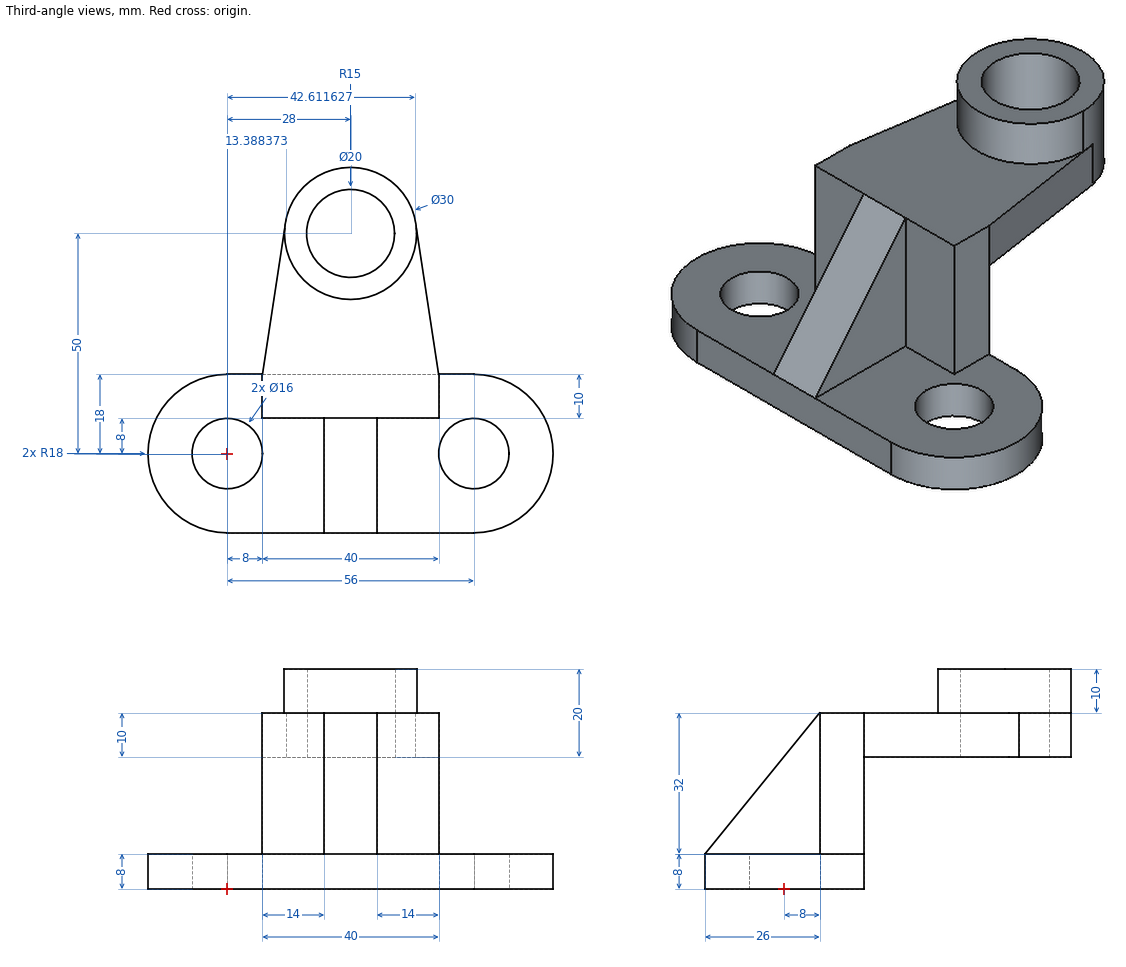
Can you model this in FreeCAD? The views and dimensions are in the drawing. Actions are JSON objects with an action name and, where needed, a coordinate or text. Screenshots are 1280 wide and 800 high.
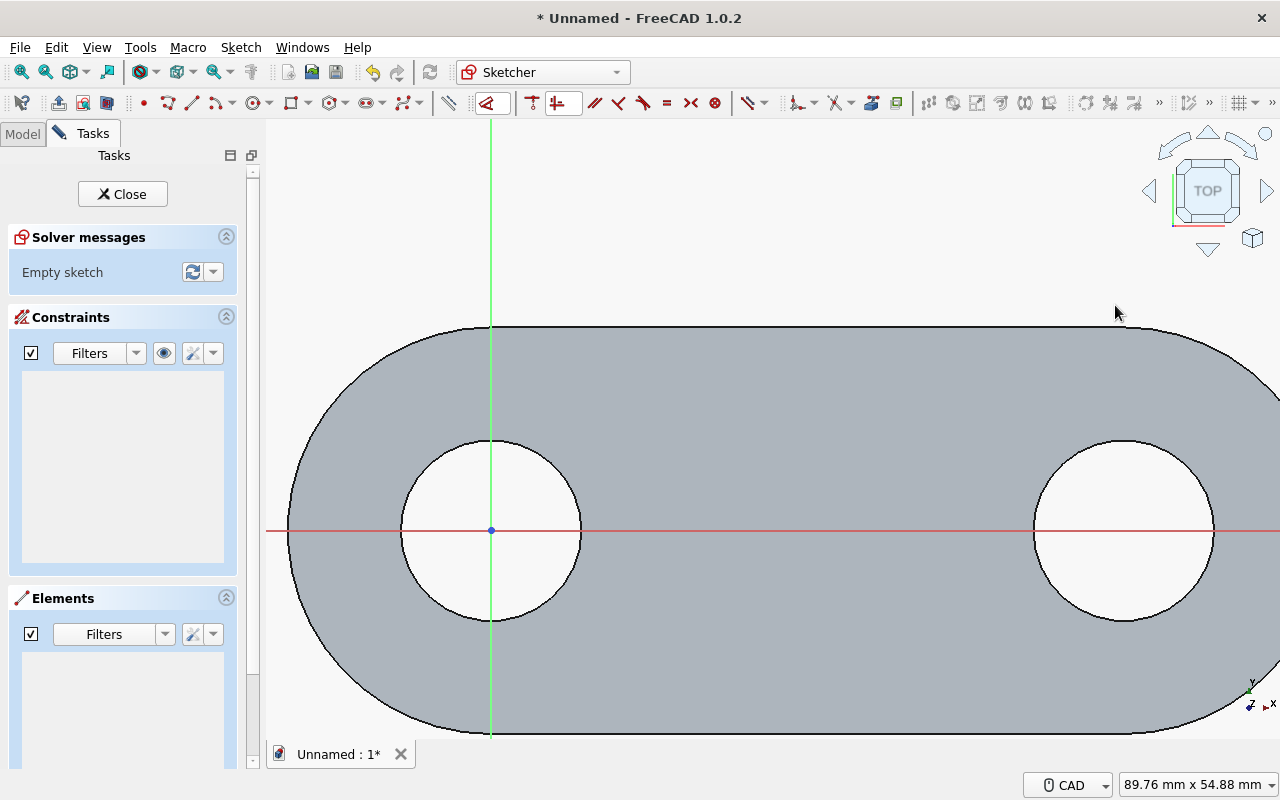
{"action": "left_click", "coordinate": [292, 104]}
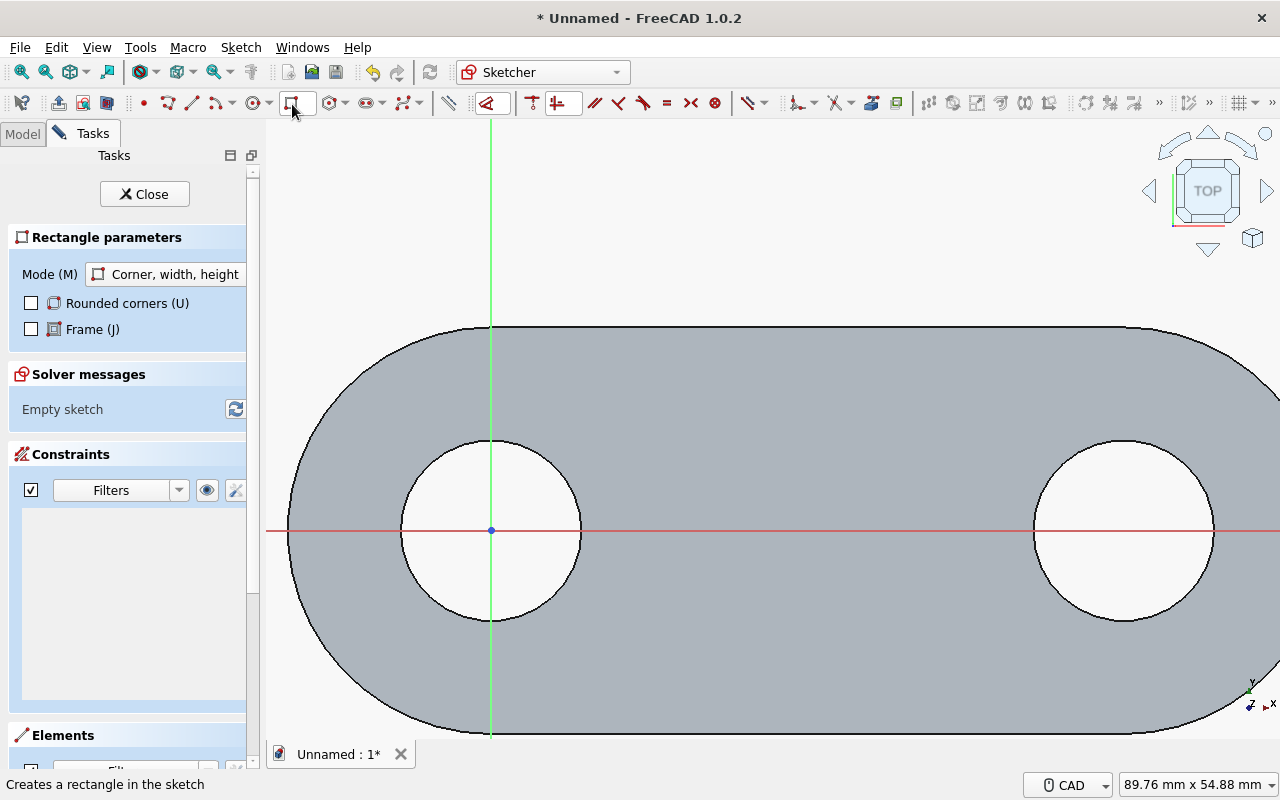
{"action": "left_click", "coordinate": [582, 327]}
{"action": "mouse_move", "coordinate": [1033, 440]}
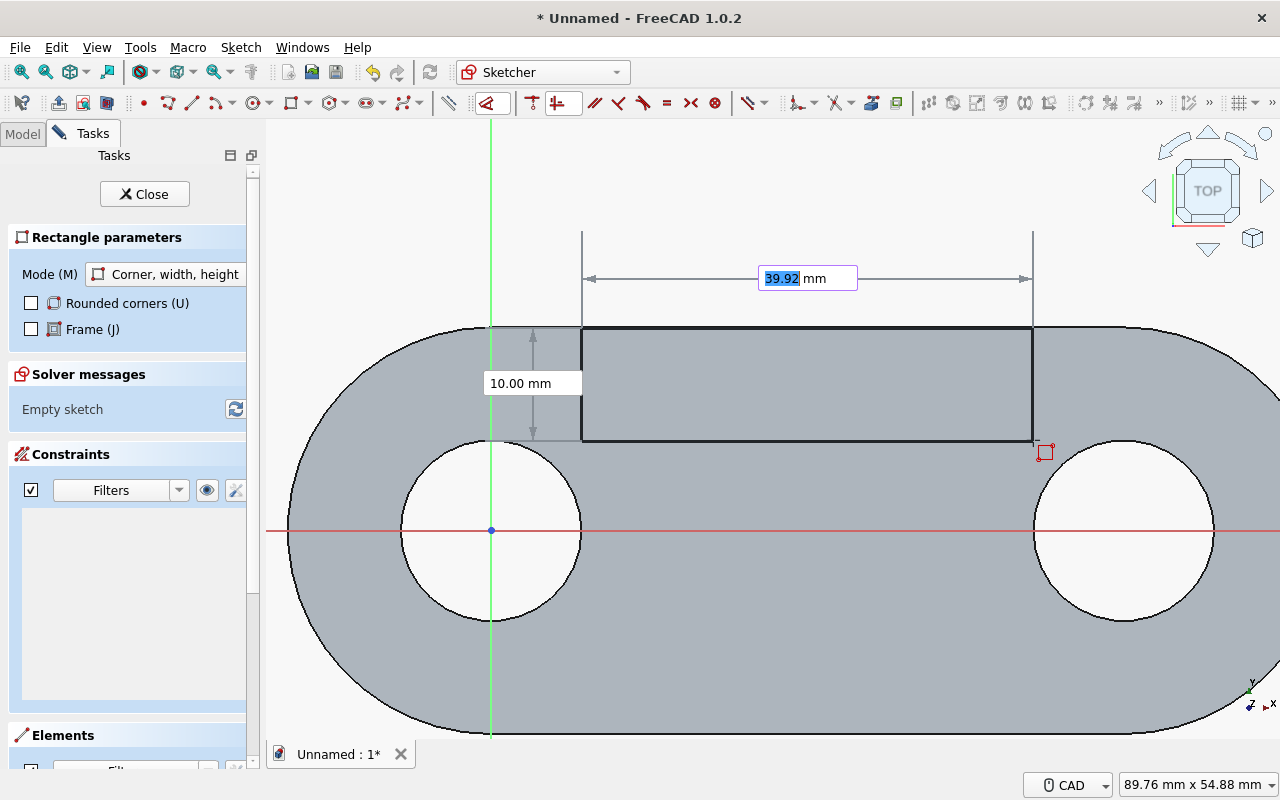
{"action": "type", "text": "40"}
{"action": "key", "text": "Tab"}
{"action": "type", "text": "10"}
{"action": "key", "text": "Return"}
{"action": "key", "text": "Escape"}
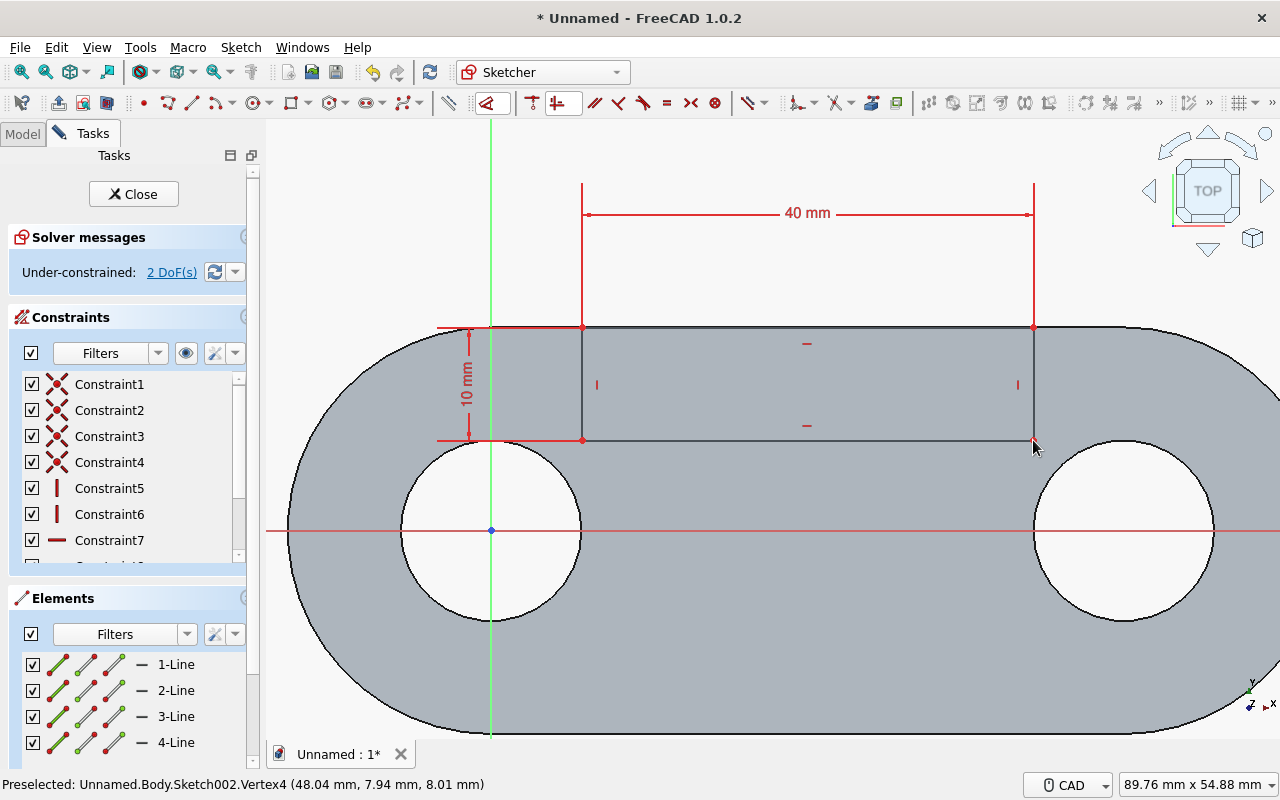
{"action": "left_click", "coordinate": [582, 328]}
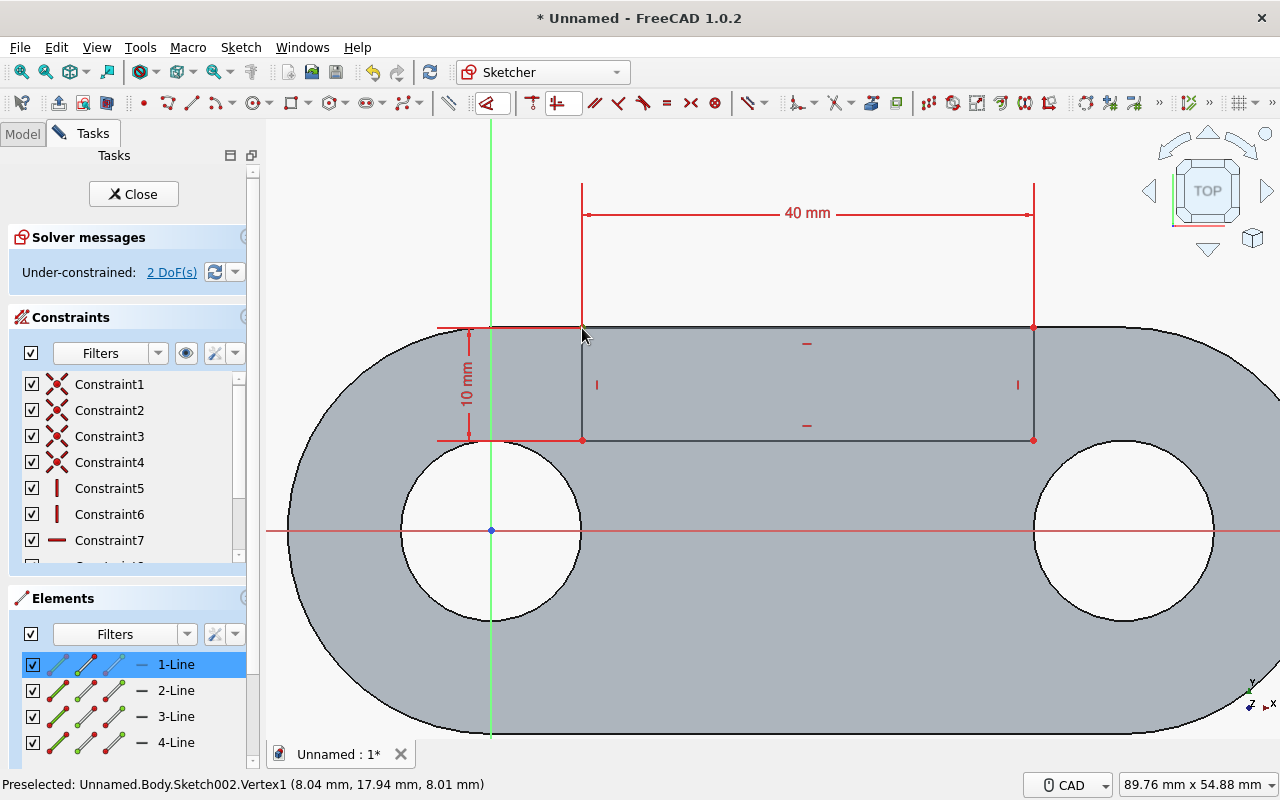
{"action": "key", "text": "l"}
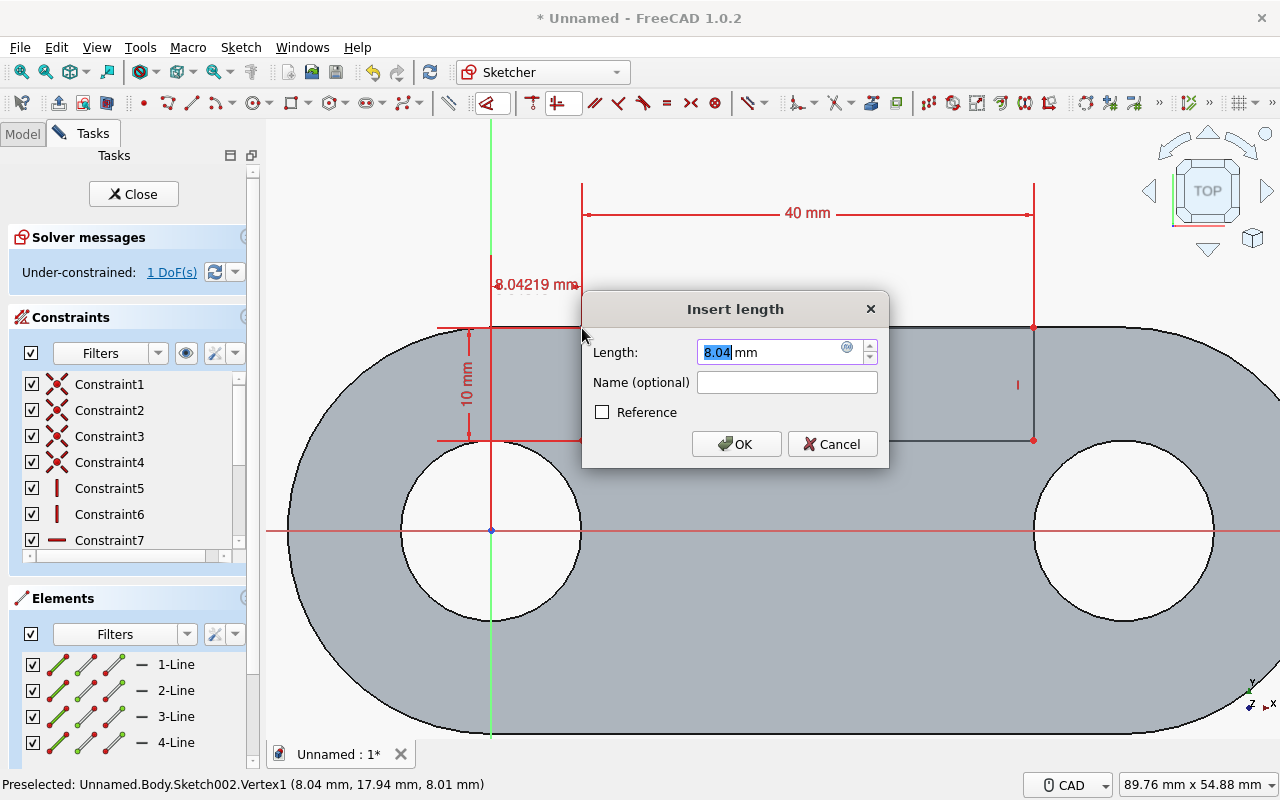
{"action": "type", "text": "8"}
{"action": "key", "text": "Return"}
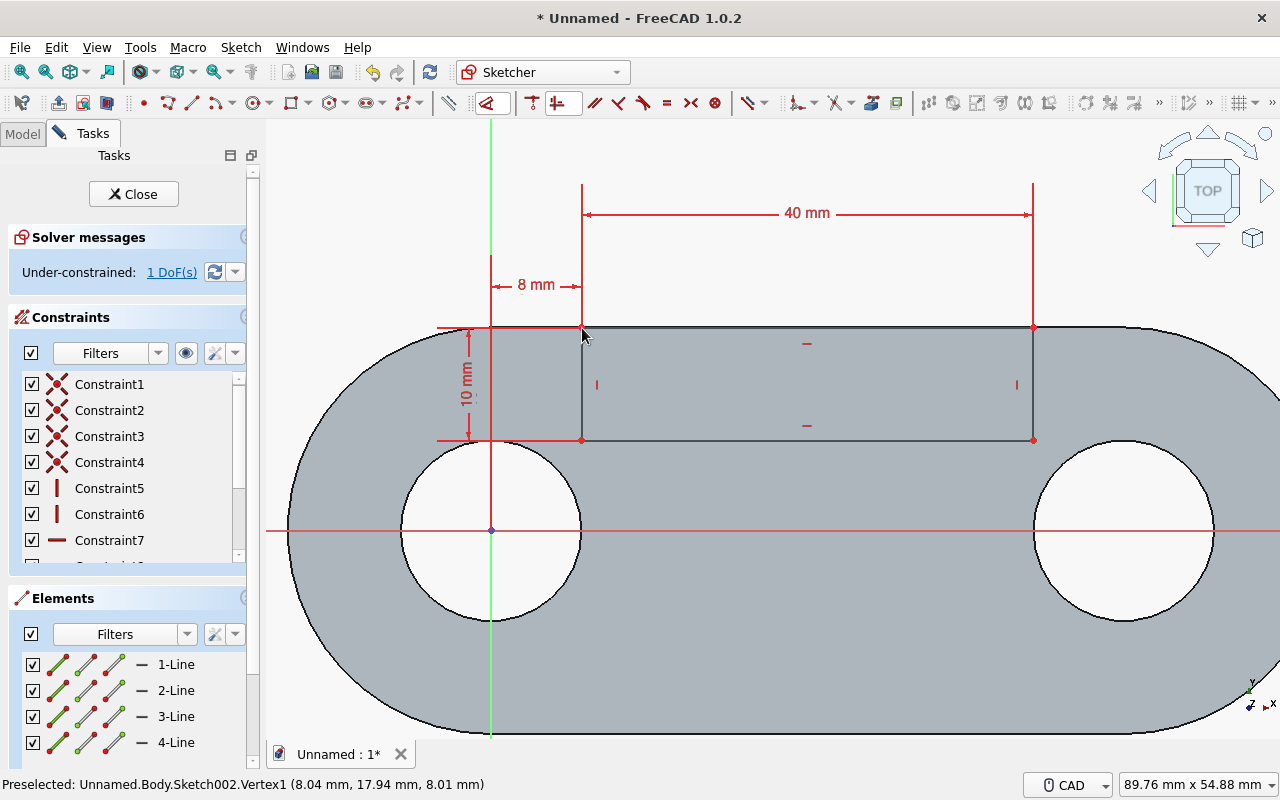
{"action": "left_click", "coordinate": [582, 441]}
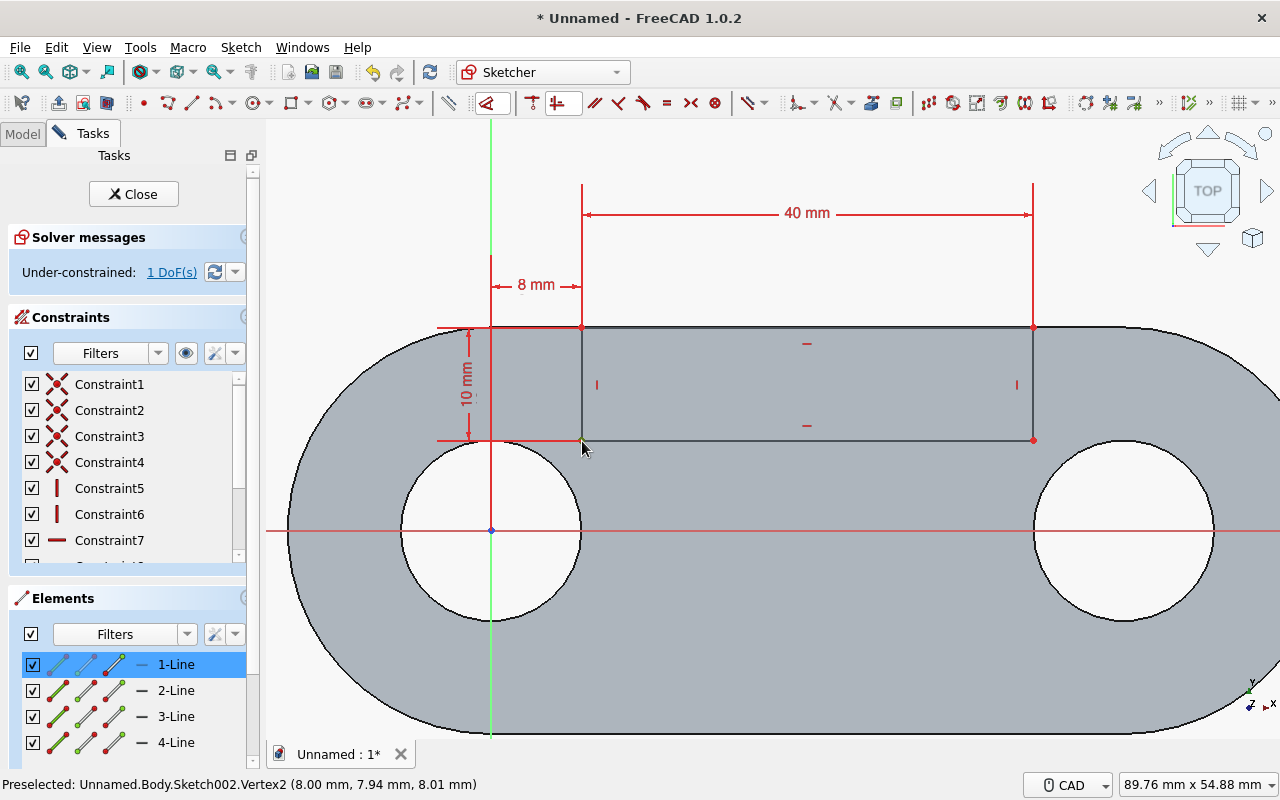
{"action": "key", "text": "i"}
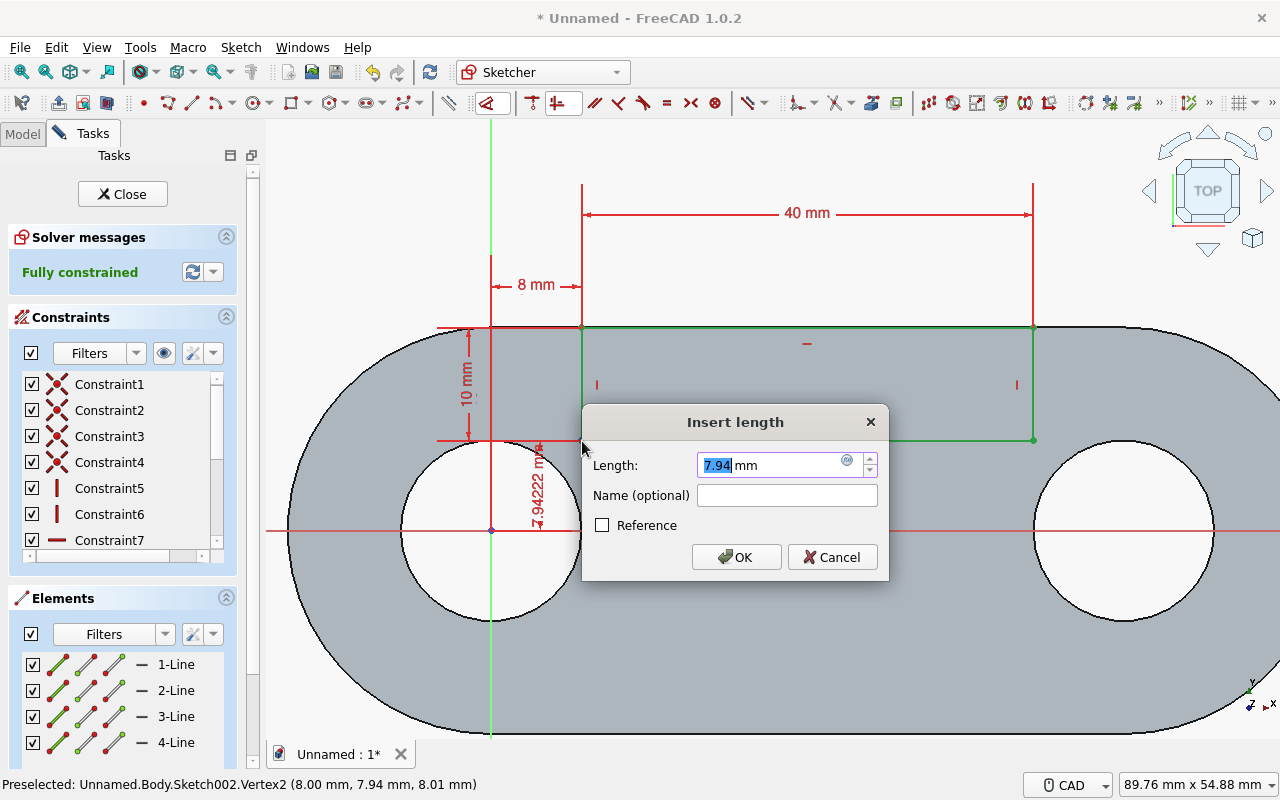
{"action": "type", "text": "8"}
{"action": "key", "text": "Return"}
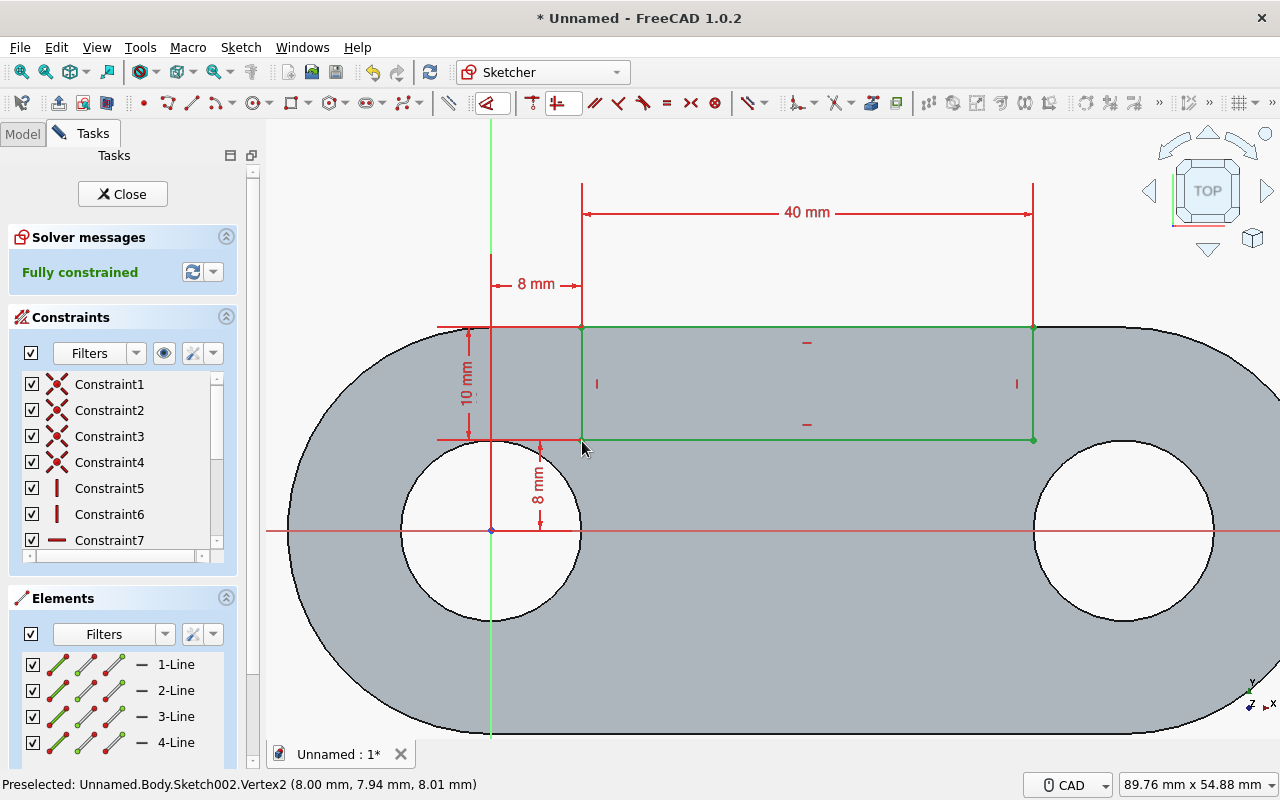
{"action": "left_click", "coordinate": [123, 194]}